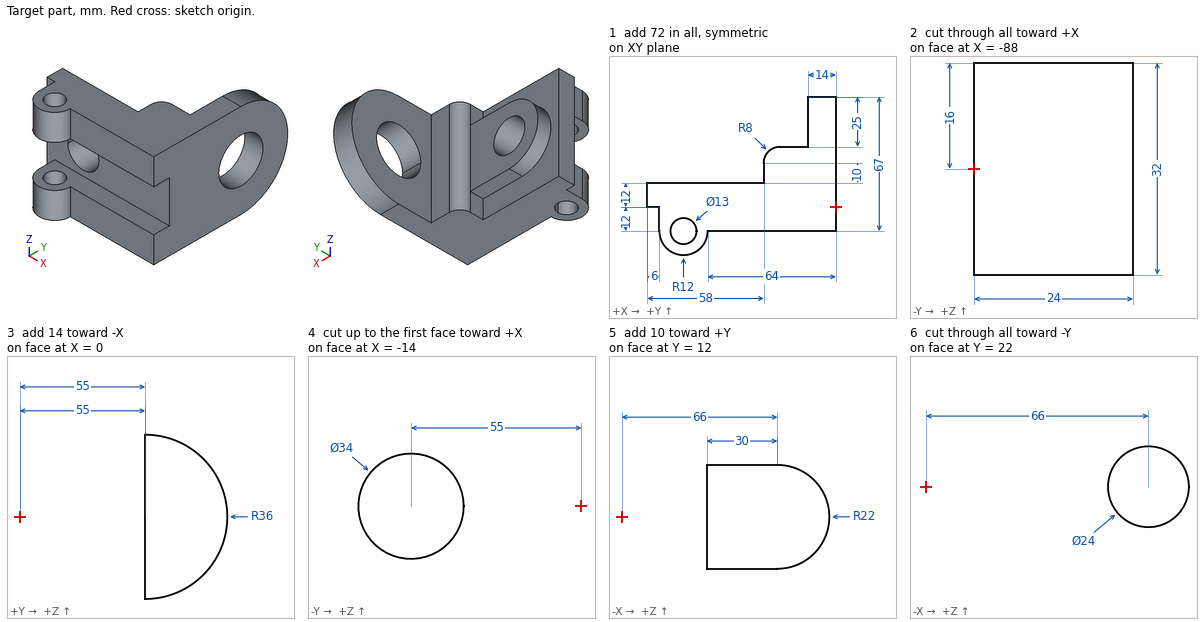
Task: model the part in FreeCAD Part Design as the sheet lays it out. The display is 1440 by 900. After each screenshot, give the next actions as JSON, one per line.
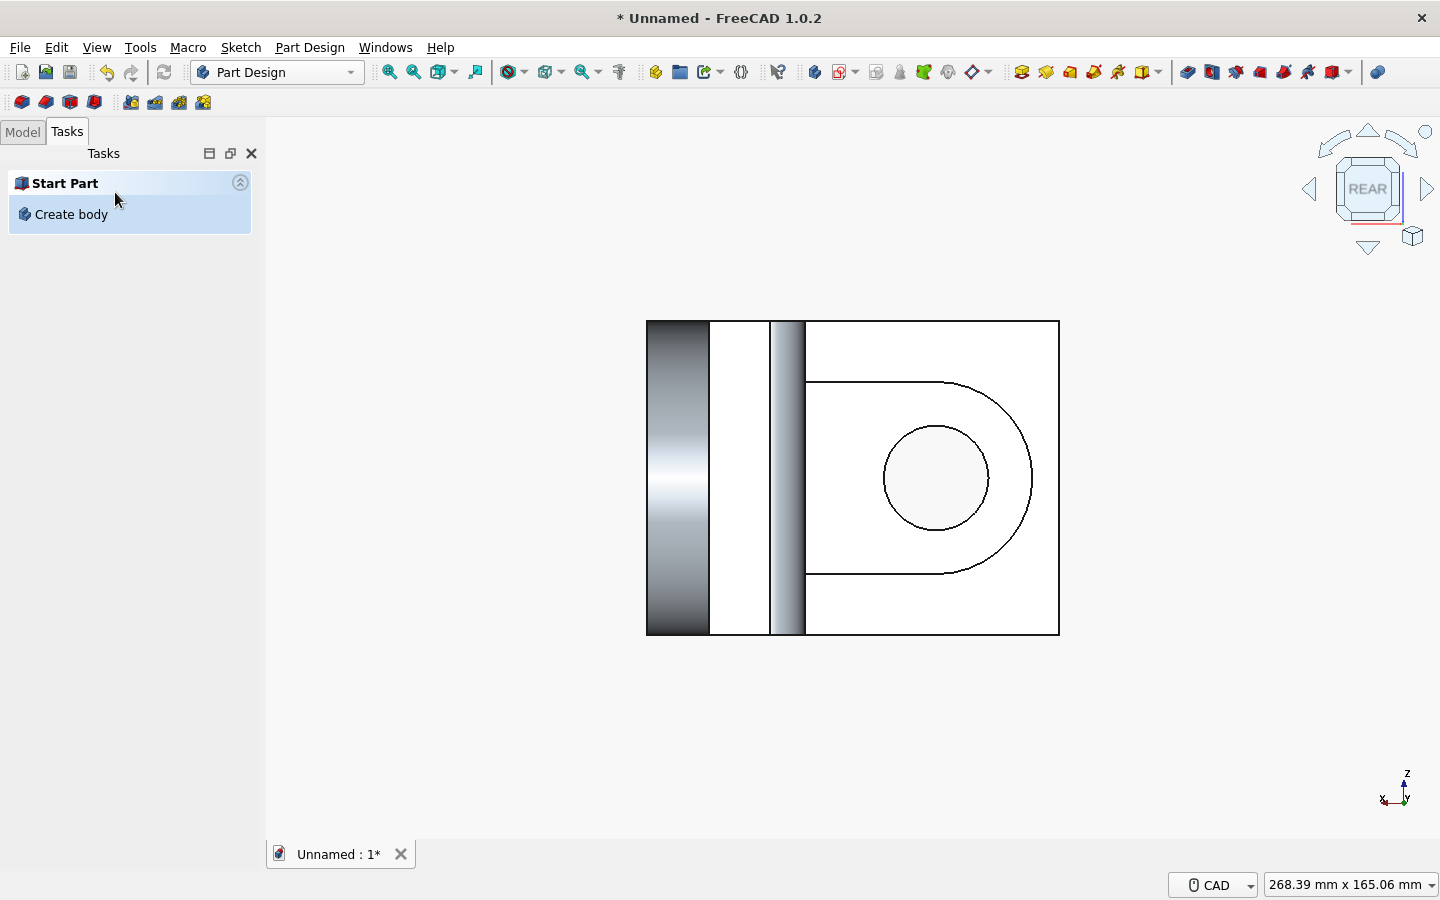
{"action": "key", "text": "0"}